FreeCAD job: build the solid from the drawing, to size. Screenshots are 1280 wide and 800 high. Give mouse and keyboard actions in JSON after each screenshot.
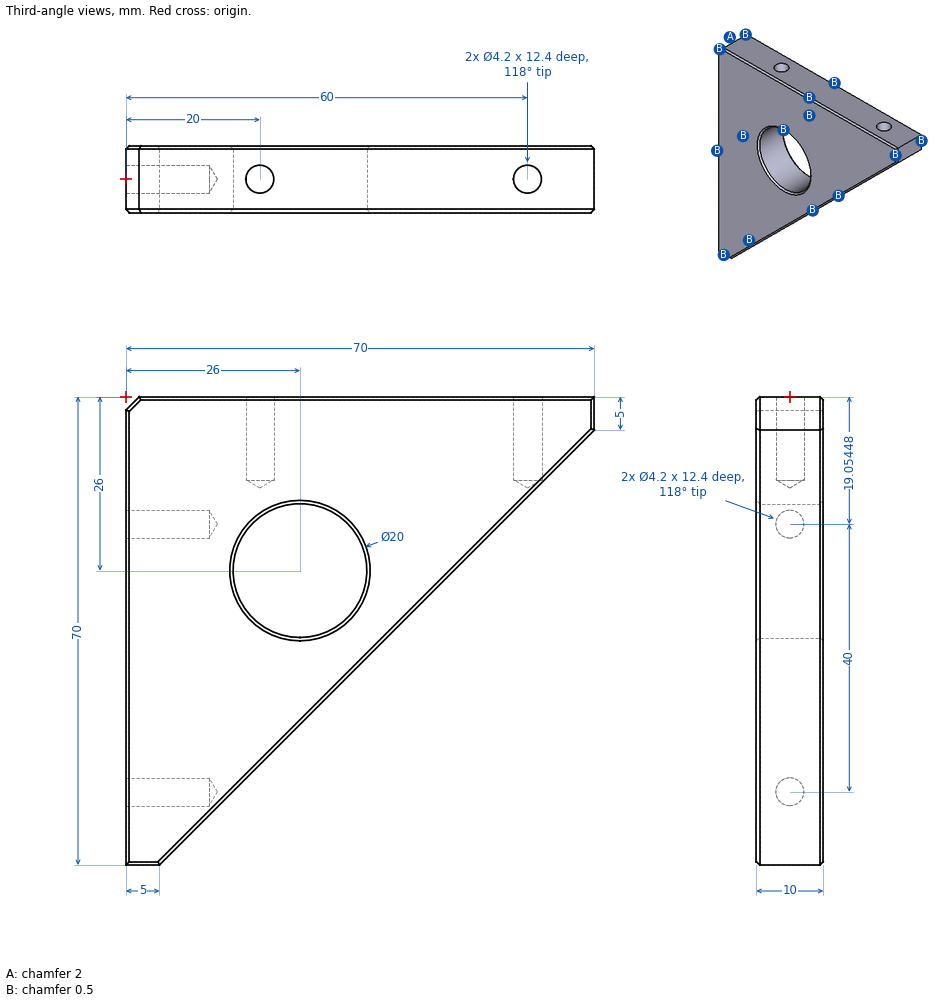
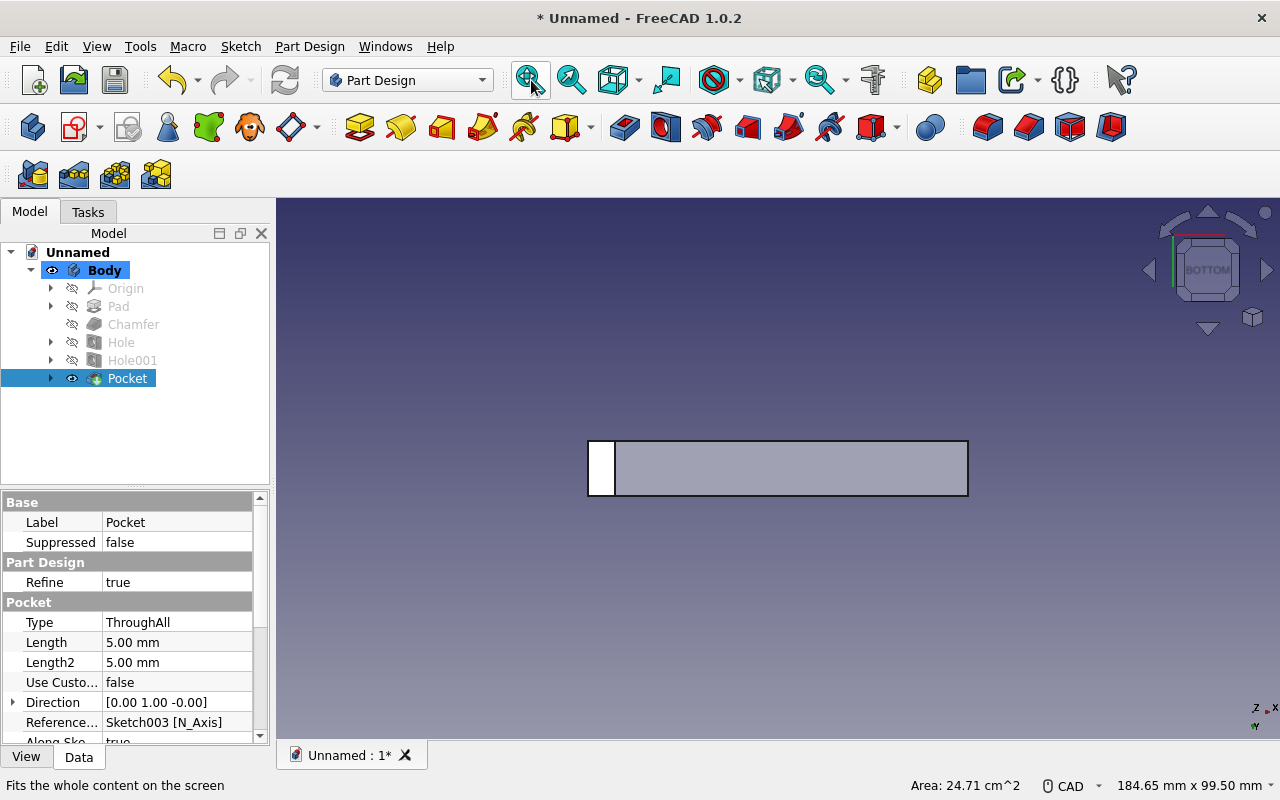
{"action": "key", "text": "4"}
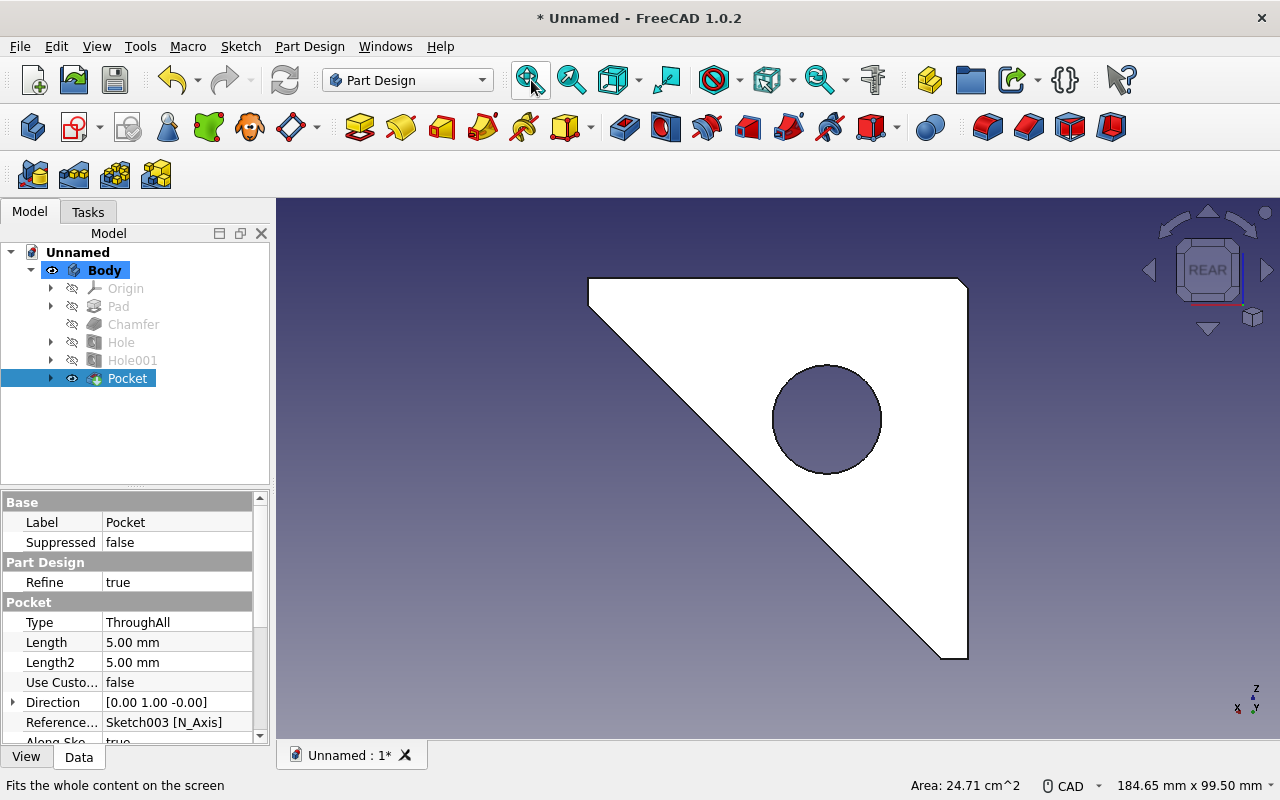
{"action": "left_click", "coordinate": [887, 522], "text": "ctrl"}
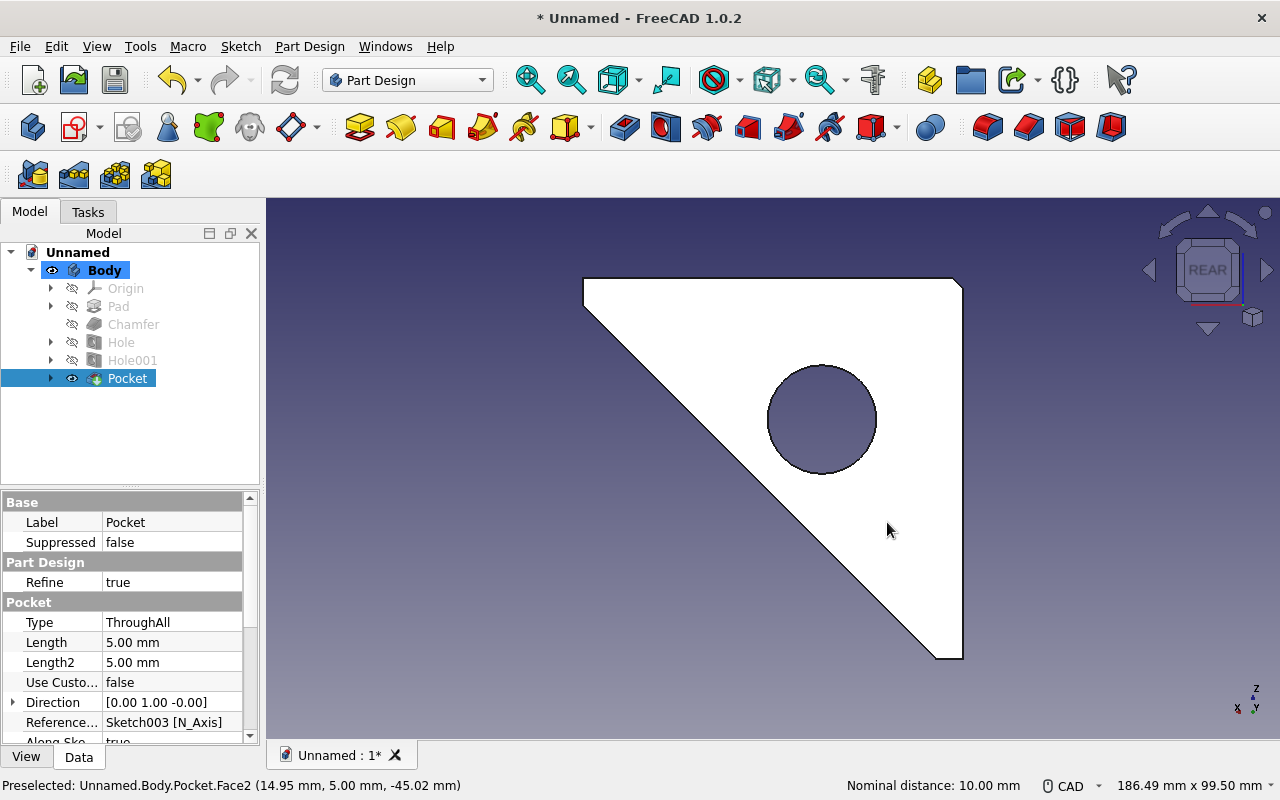
{"action": "left_click", "coordinate": [1029, 128]}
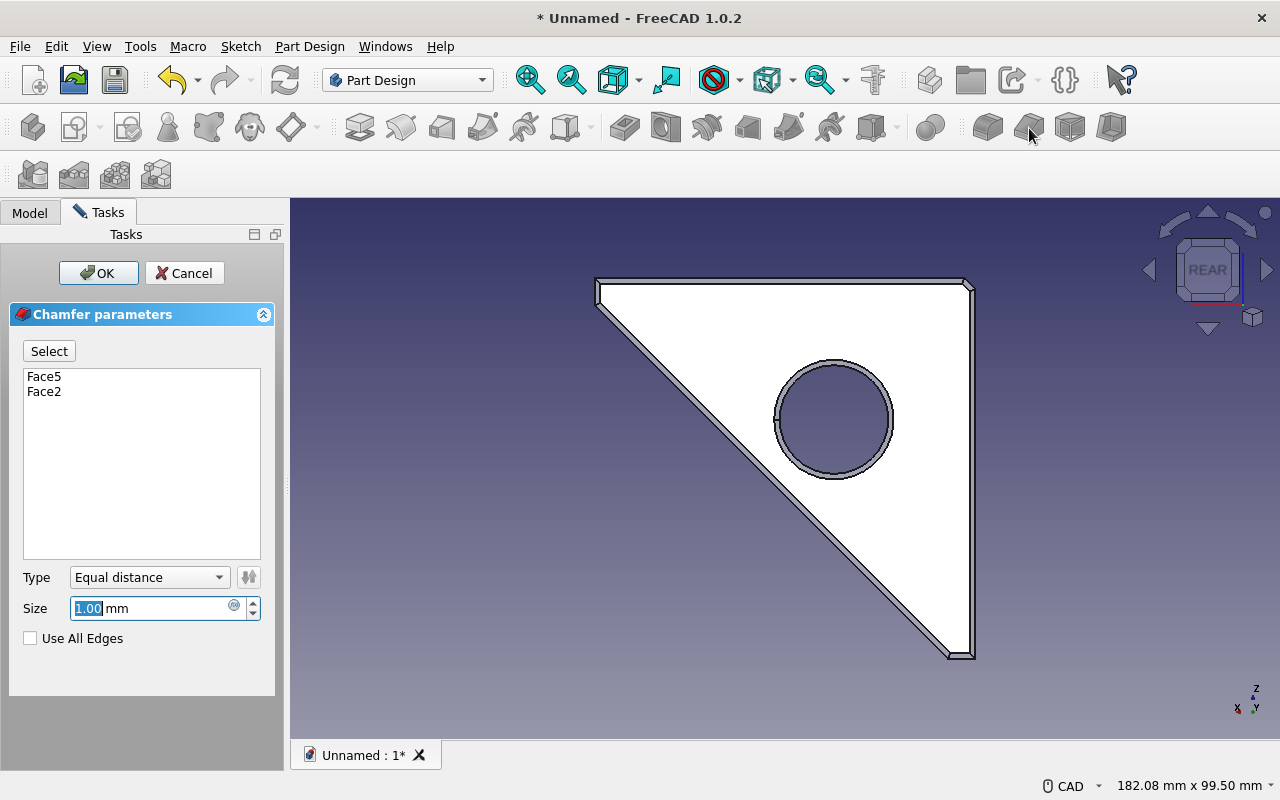
{"action": "type", "text": "0.5"}
{"action": "key", "text": "Tab"}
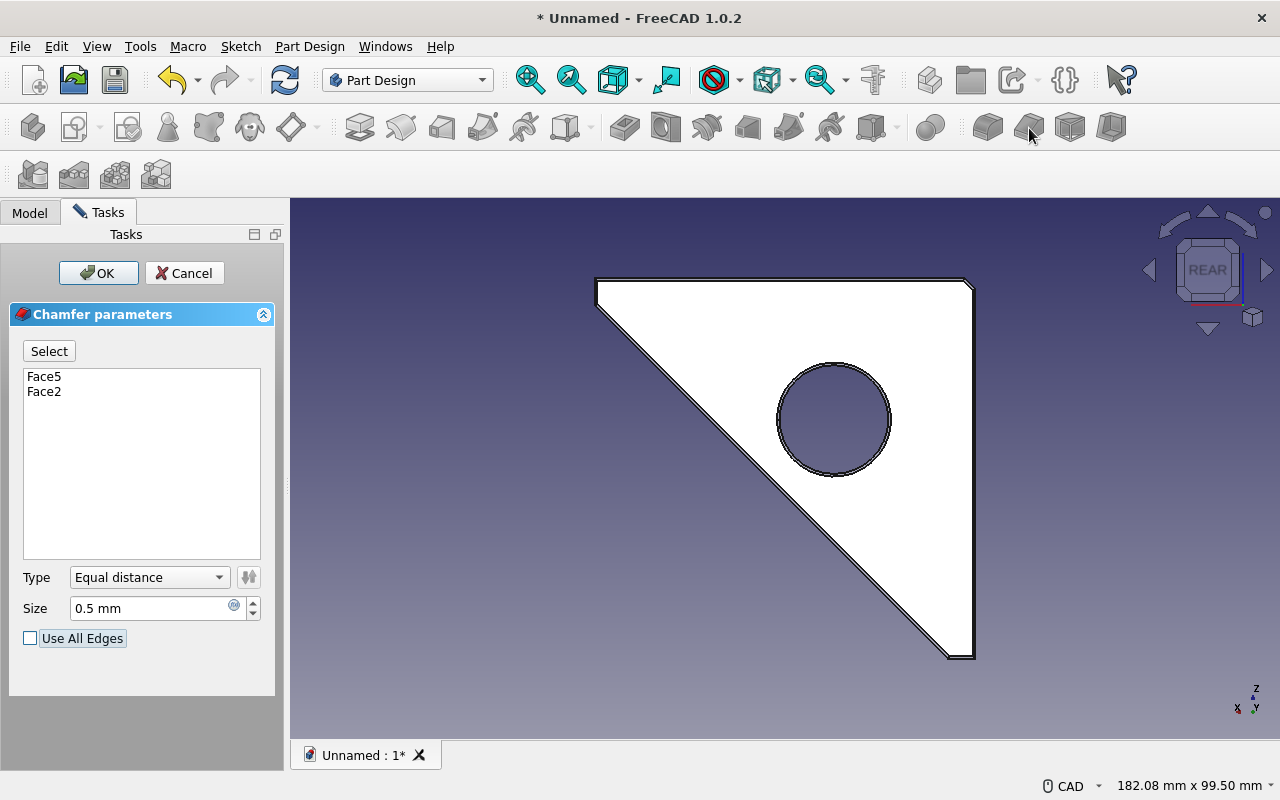
{"action": "left_click", "coordinate": [99, 273]}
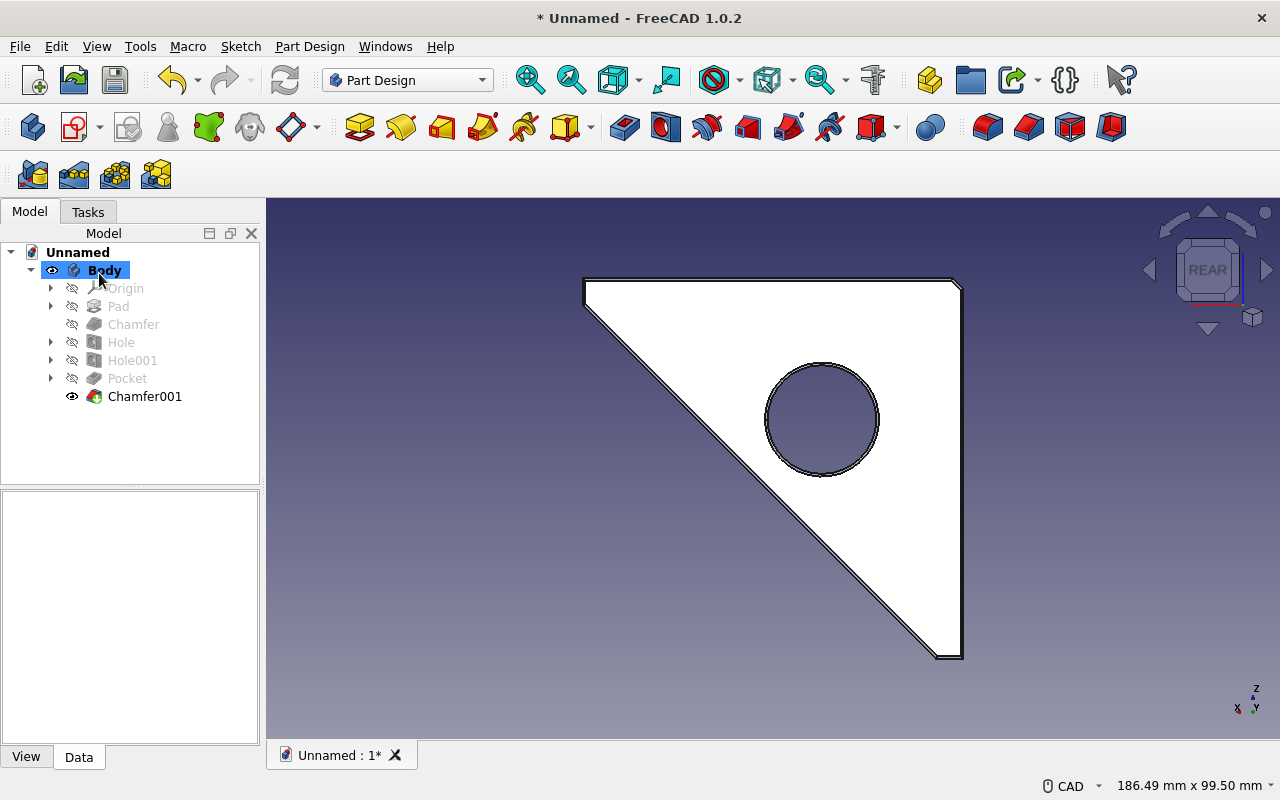
{"action": "key", "text": "0"}